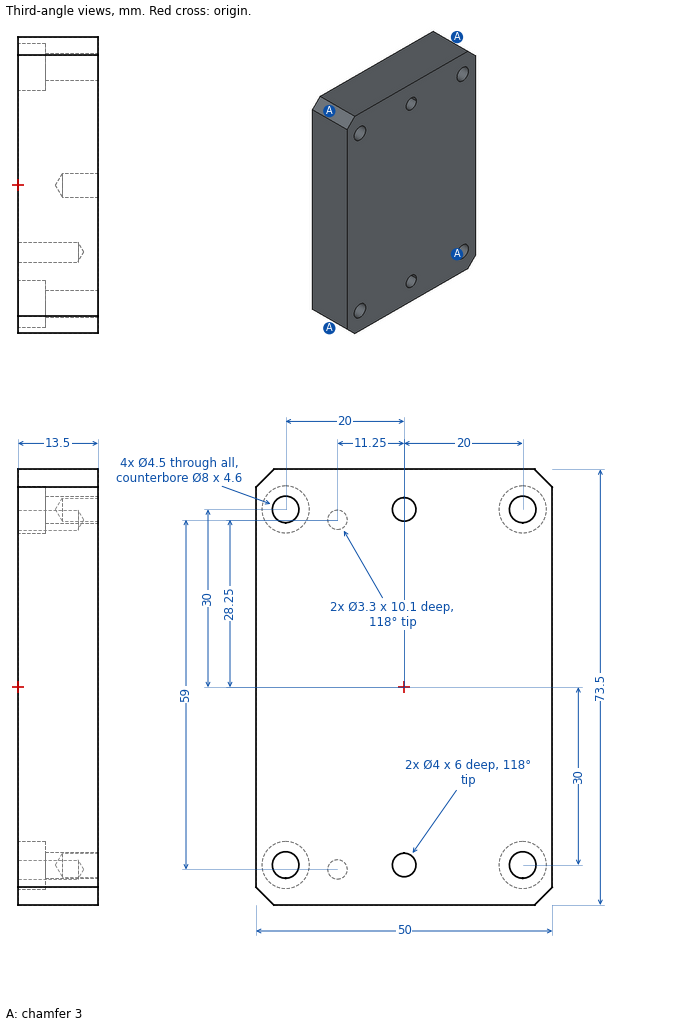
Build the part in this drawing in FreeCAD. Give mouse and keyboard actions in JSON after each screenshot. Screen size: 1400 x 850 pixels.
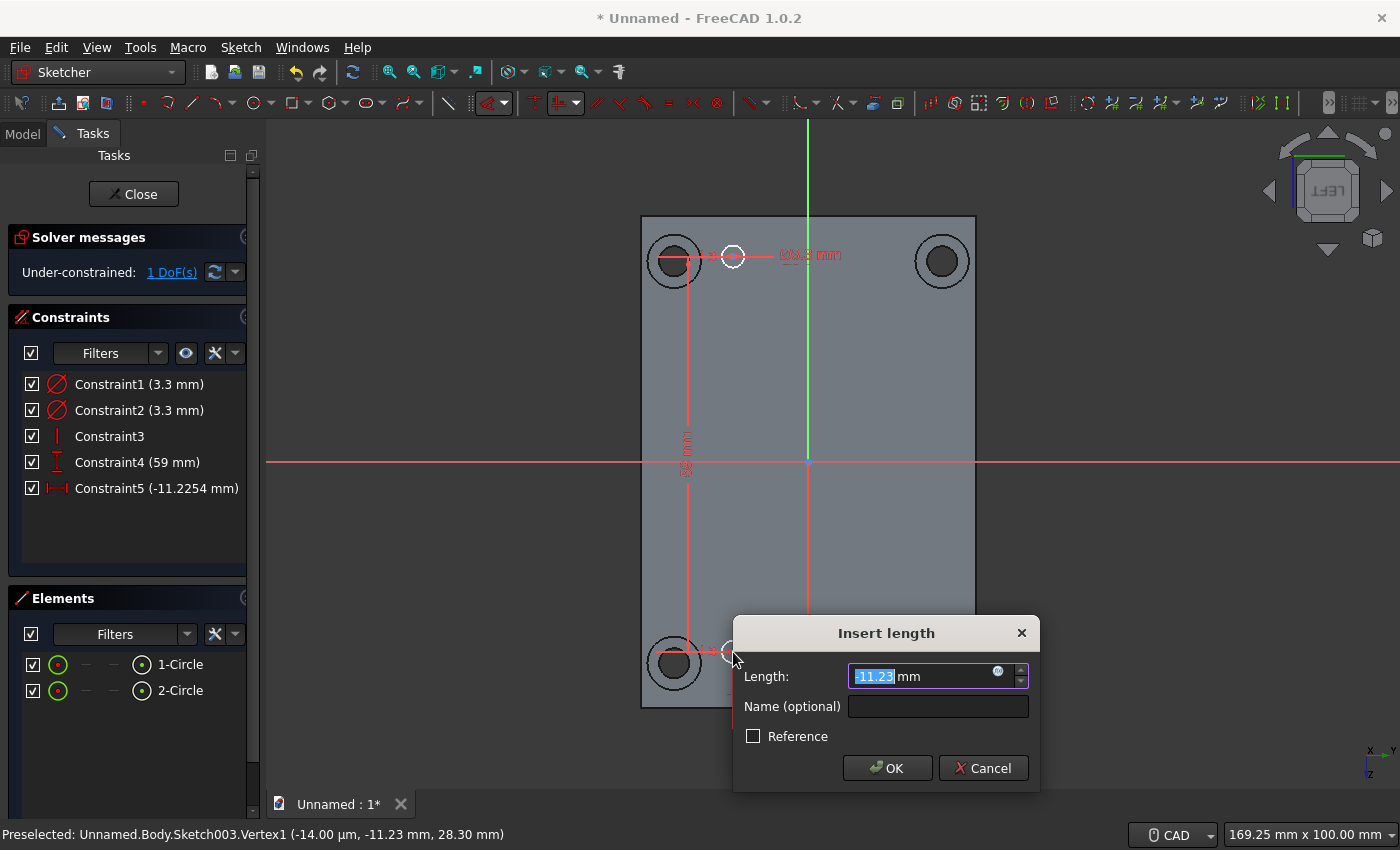
{"action": "type", "text": "-11.25"}
{"action": "key", "text": "Return"}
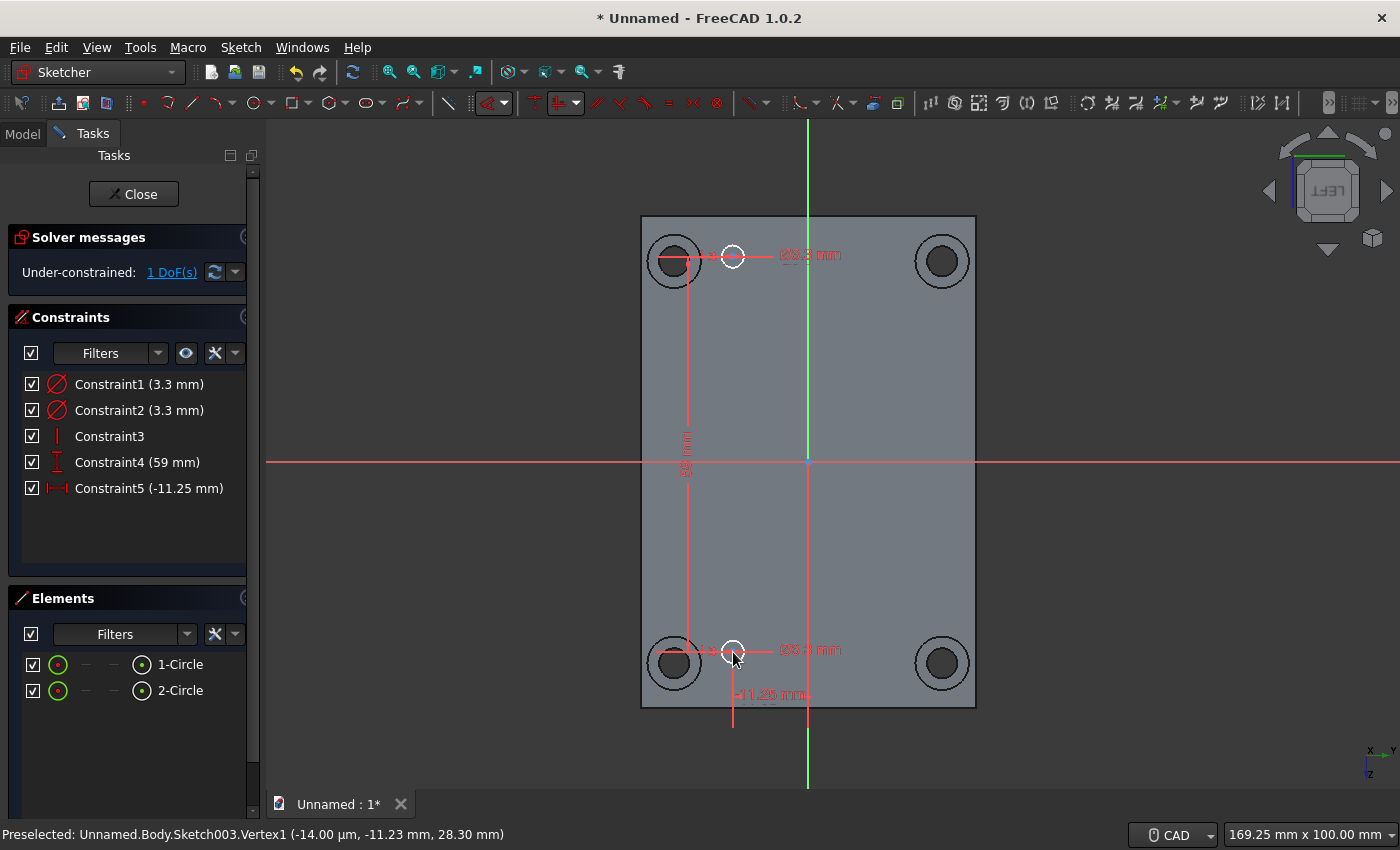
{"action": "left_click", "coordinate": [733, 652]}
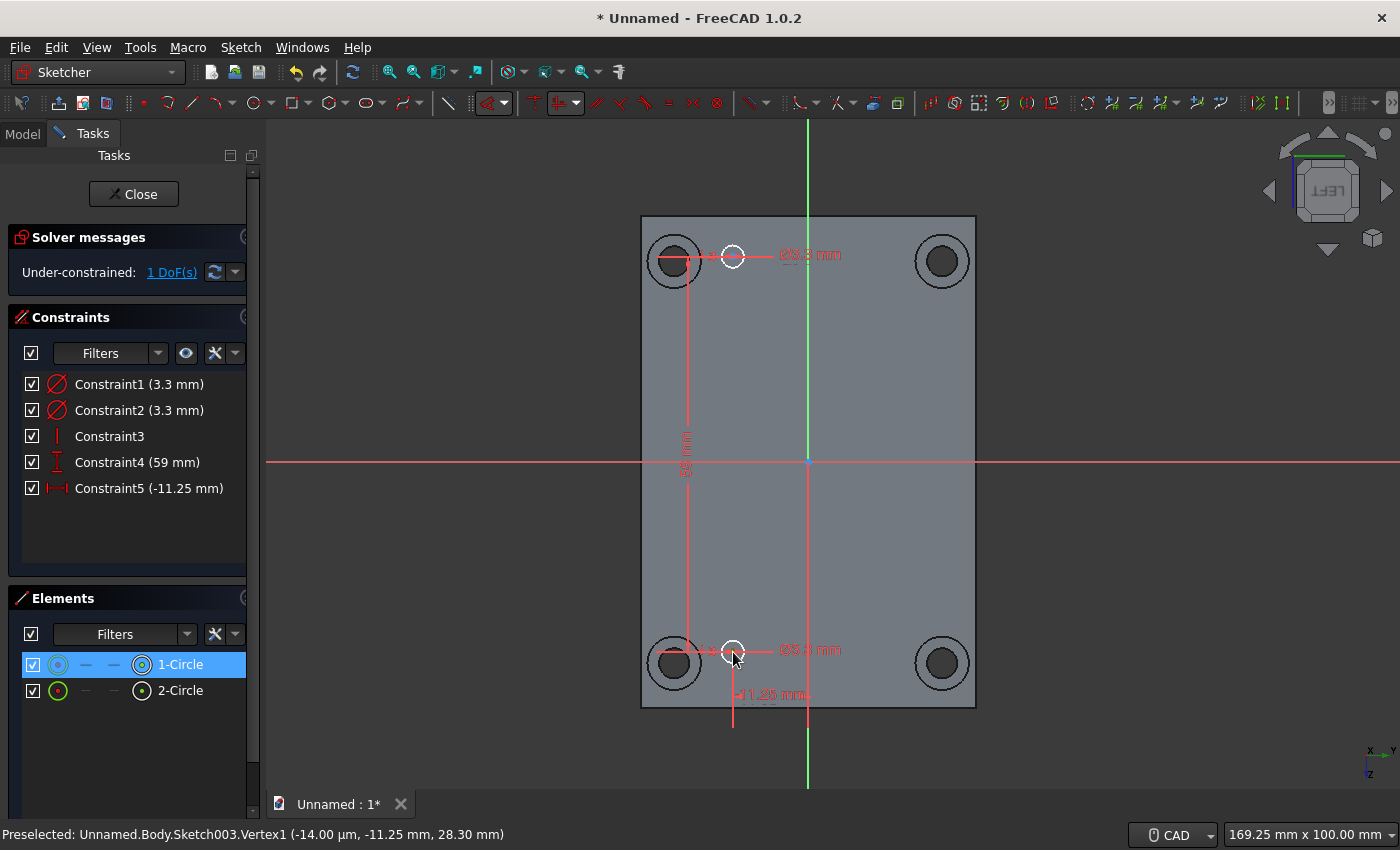
{"action": "key", "text": "i"}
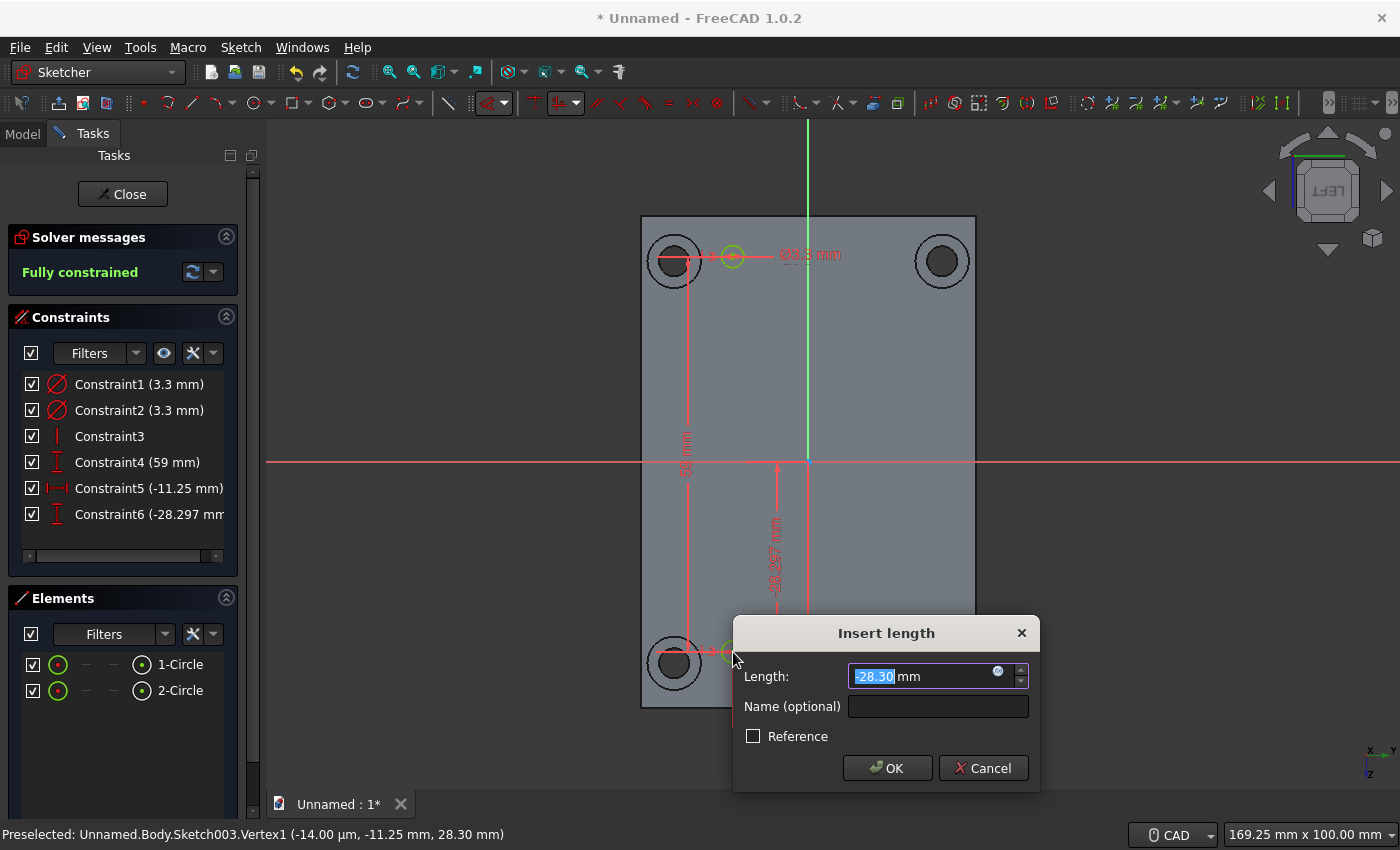
{"action": "type", "text": "-28.25"}
{"action": "key", "text": "Return"}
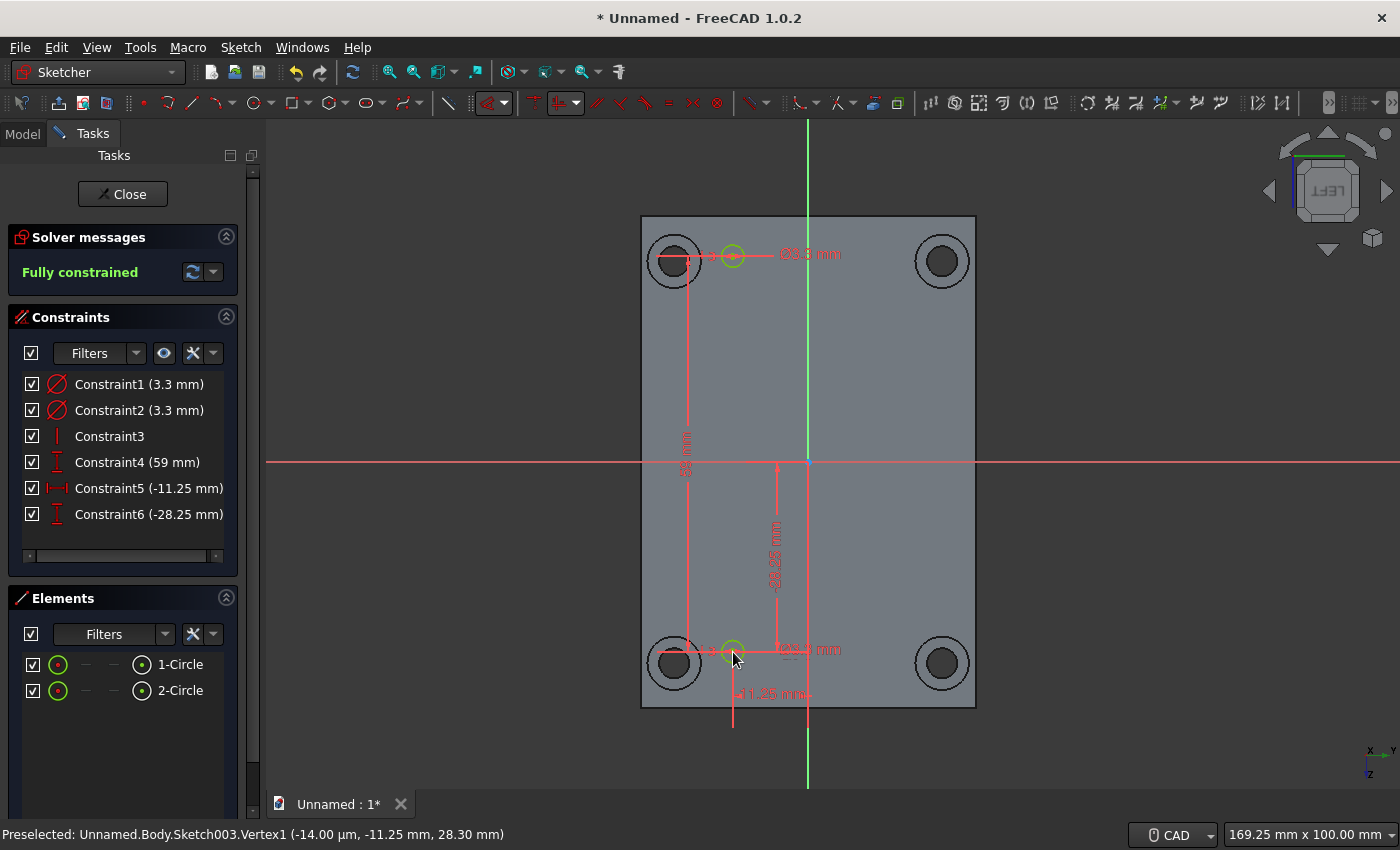
{"action": "left_click", "coordinate": [123, 194]}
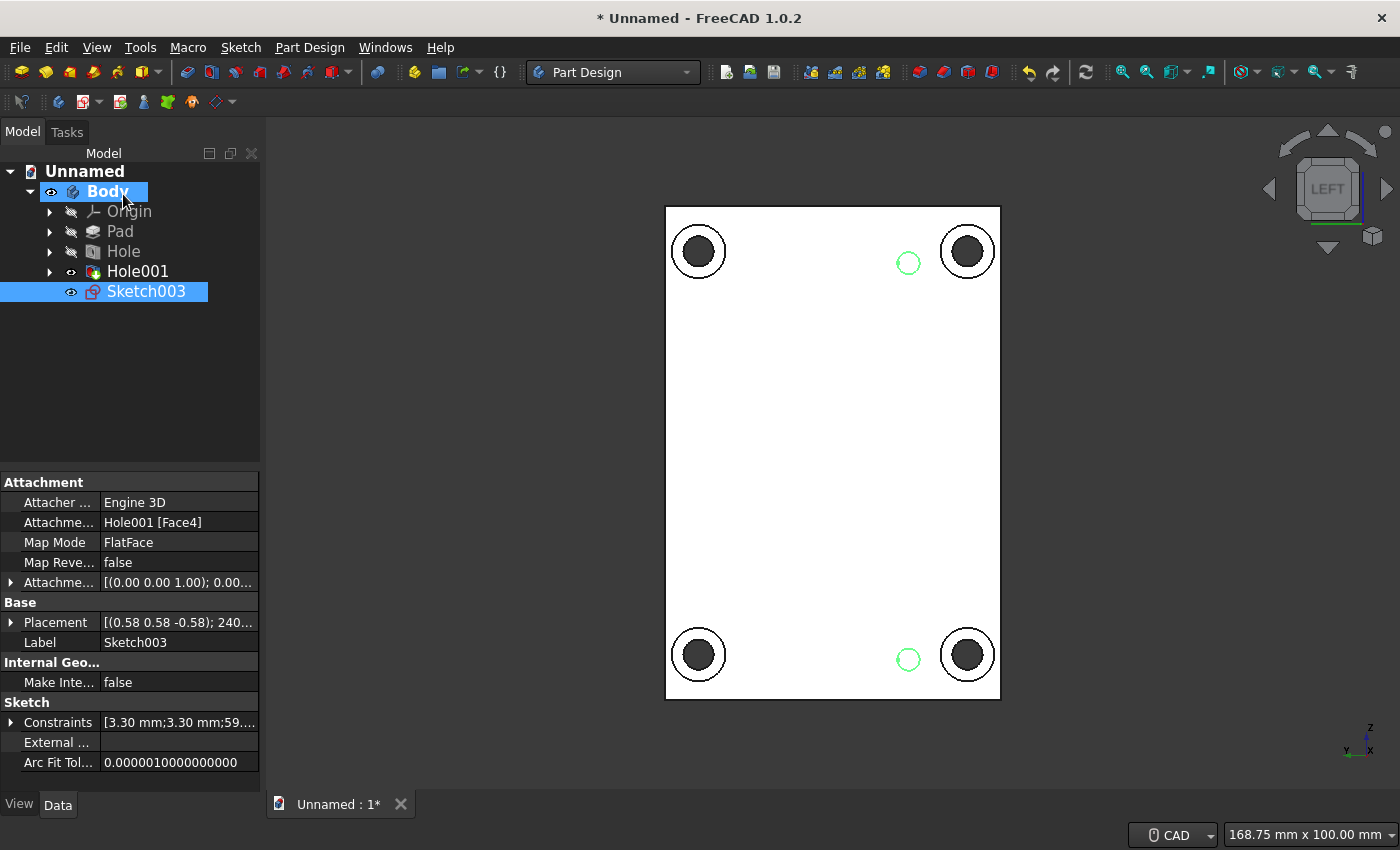
{"action": "left_click", "coordinate": [212, 72]}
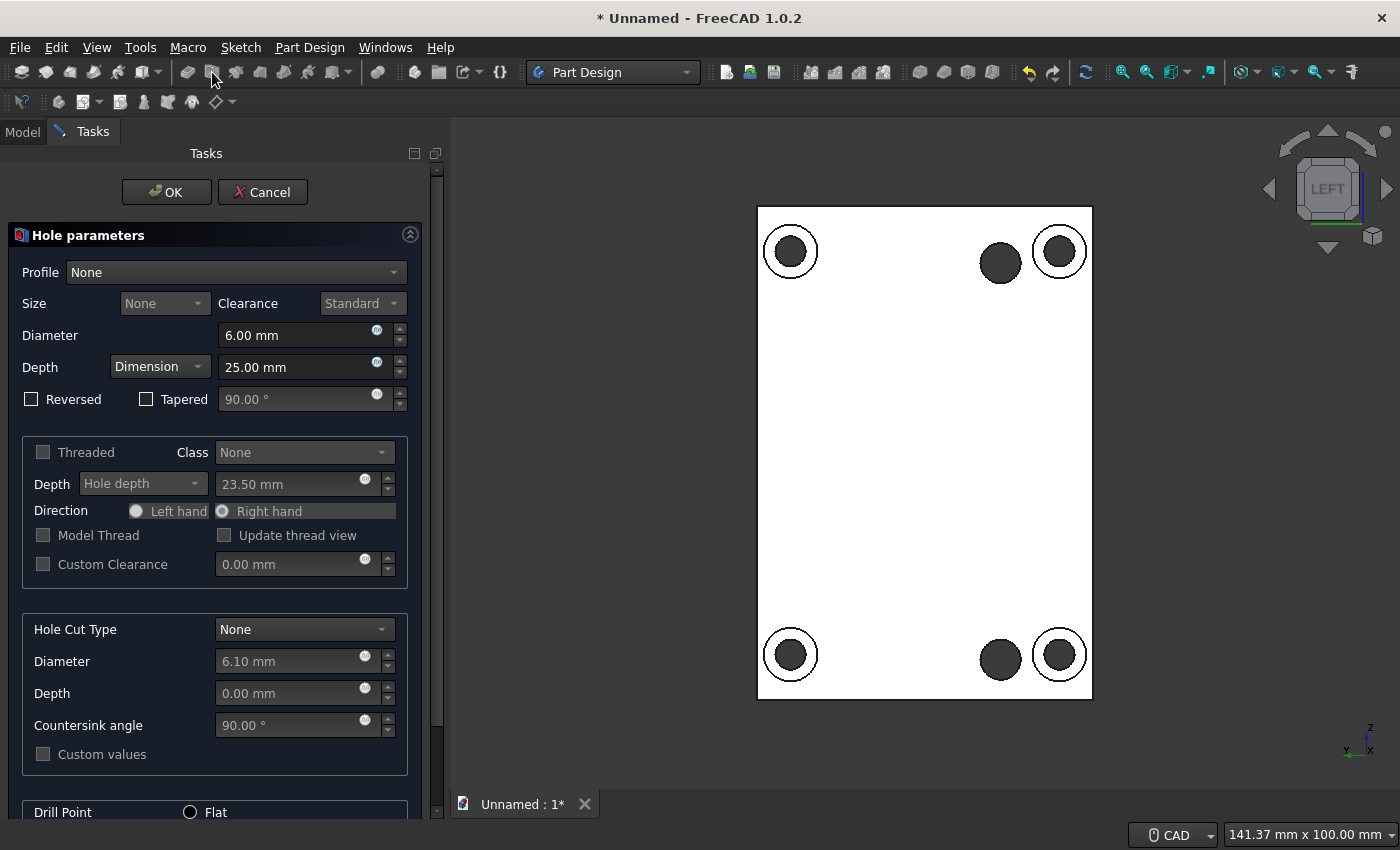
{"action": "triple_click", "coordinate": [305, 335]}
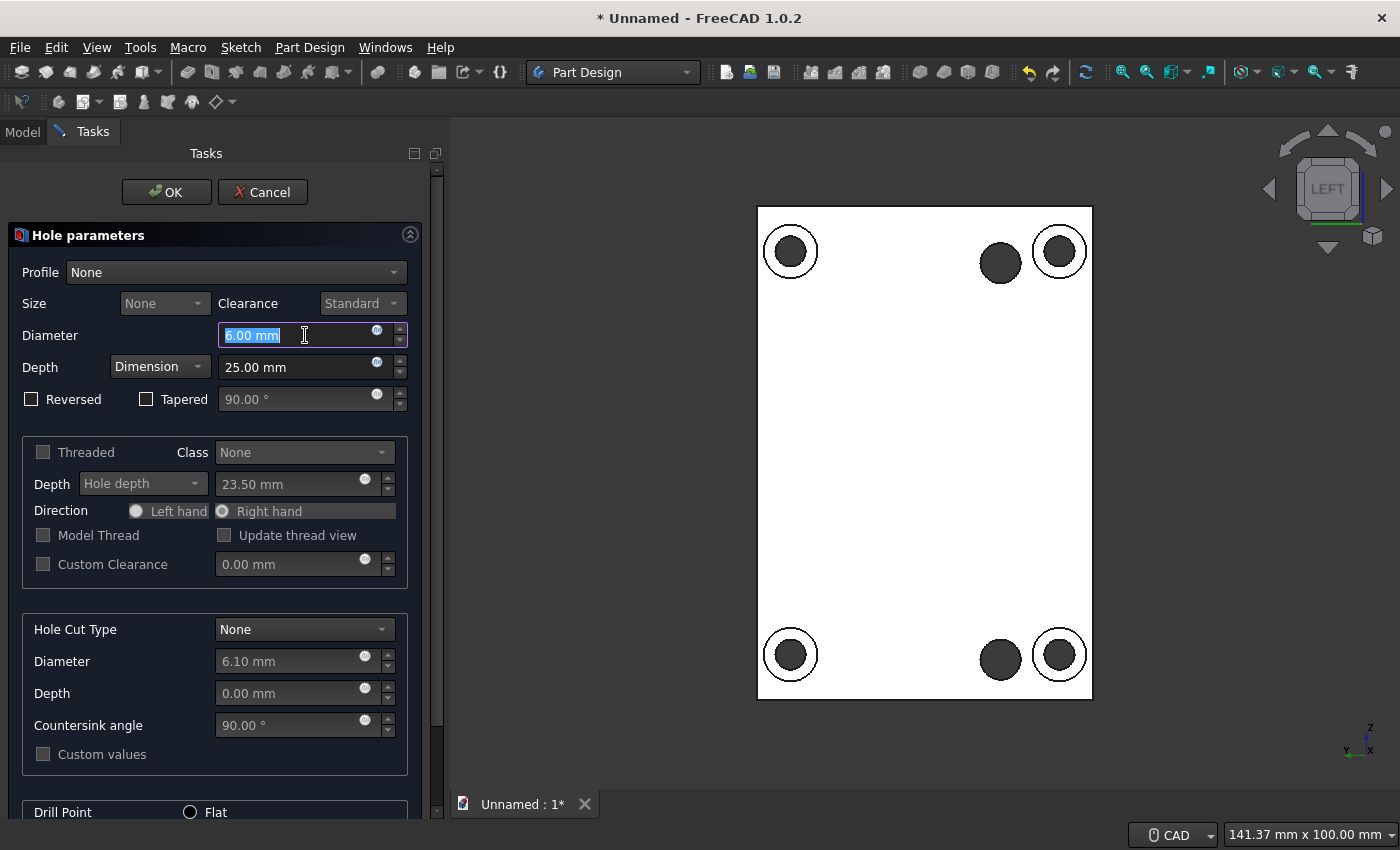
{"action": "type", "text": "3.3"}
{"action": "key", "text": "Tab"}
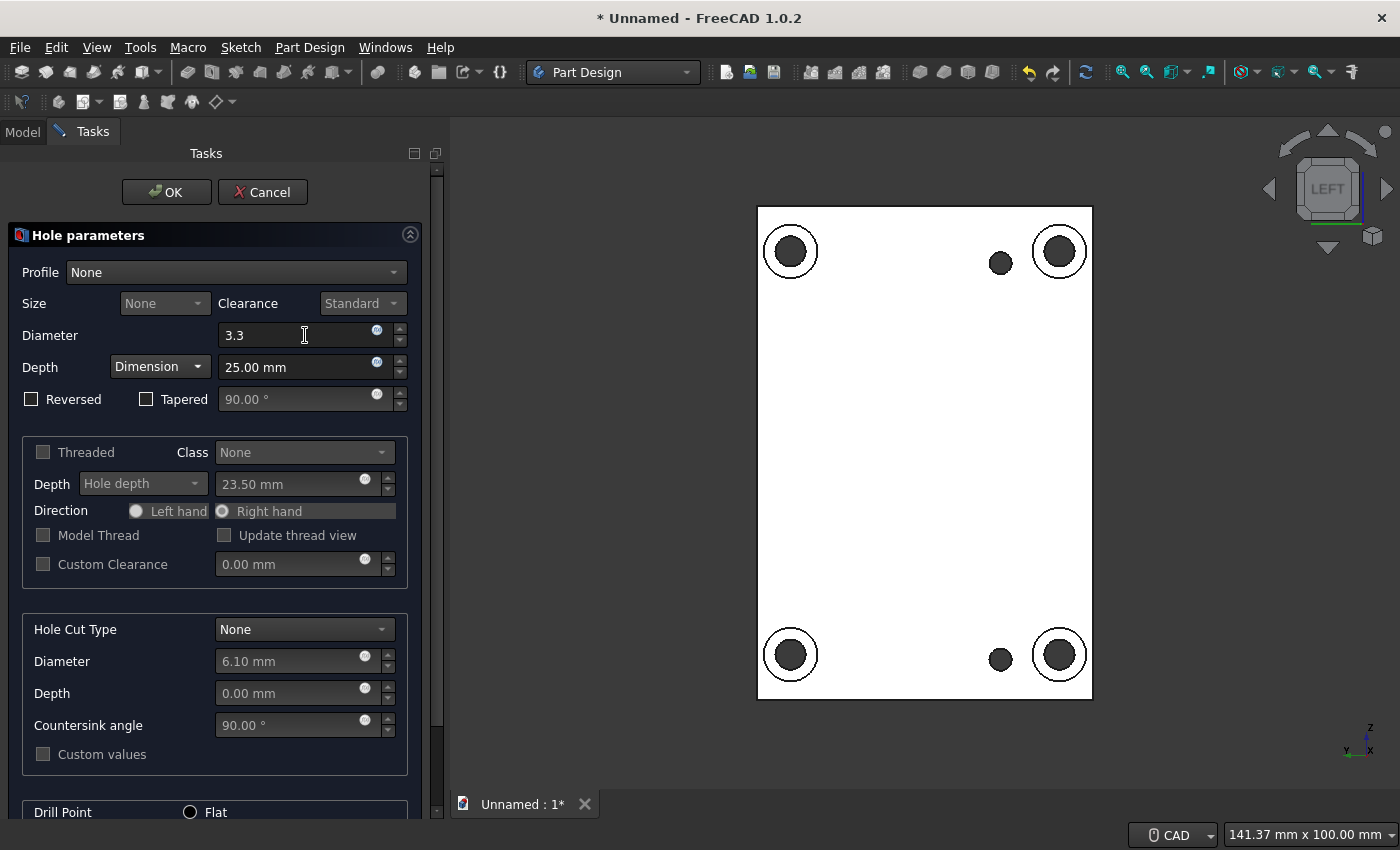
{"action": "triple_click", "coordinate": [305, 367]}